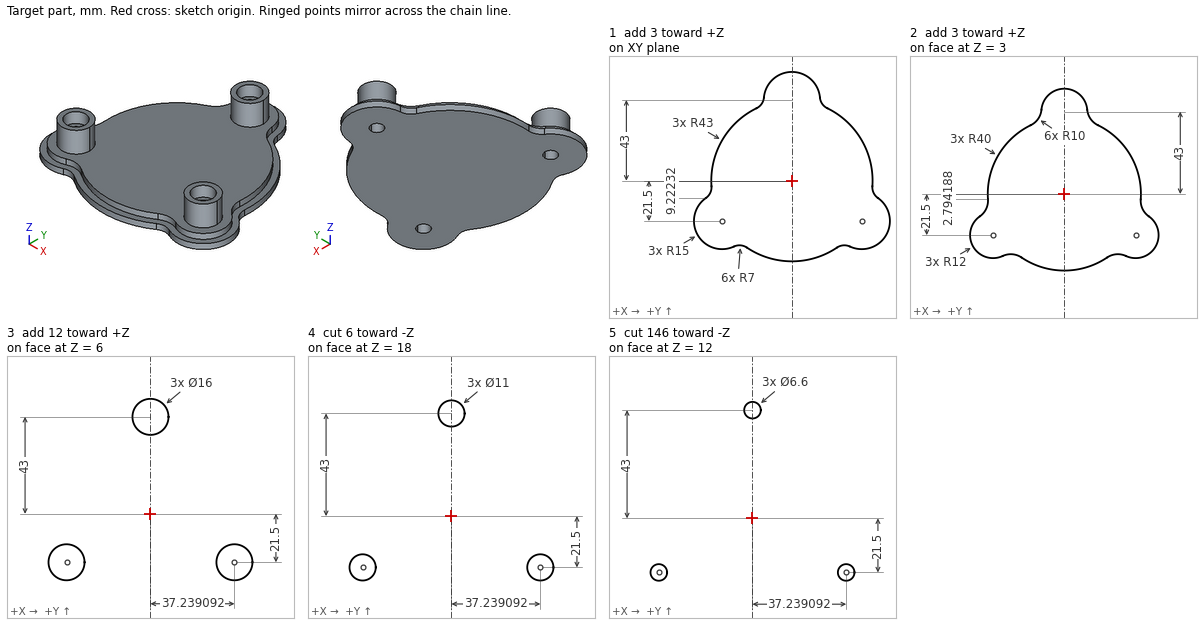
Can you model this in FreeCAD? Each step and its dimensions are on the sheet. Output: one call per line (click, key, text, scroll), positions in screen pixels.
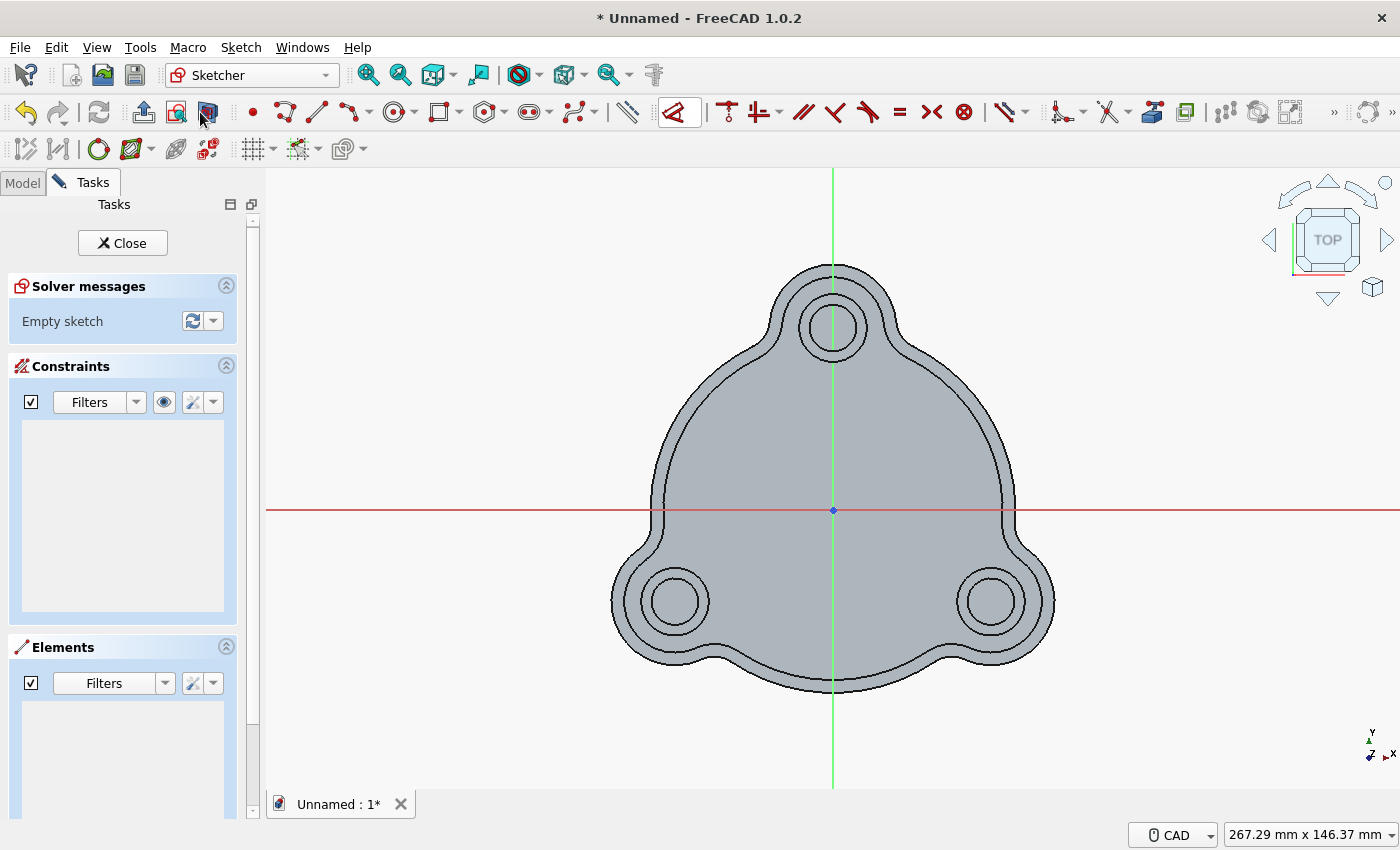
click(208, 112)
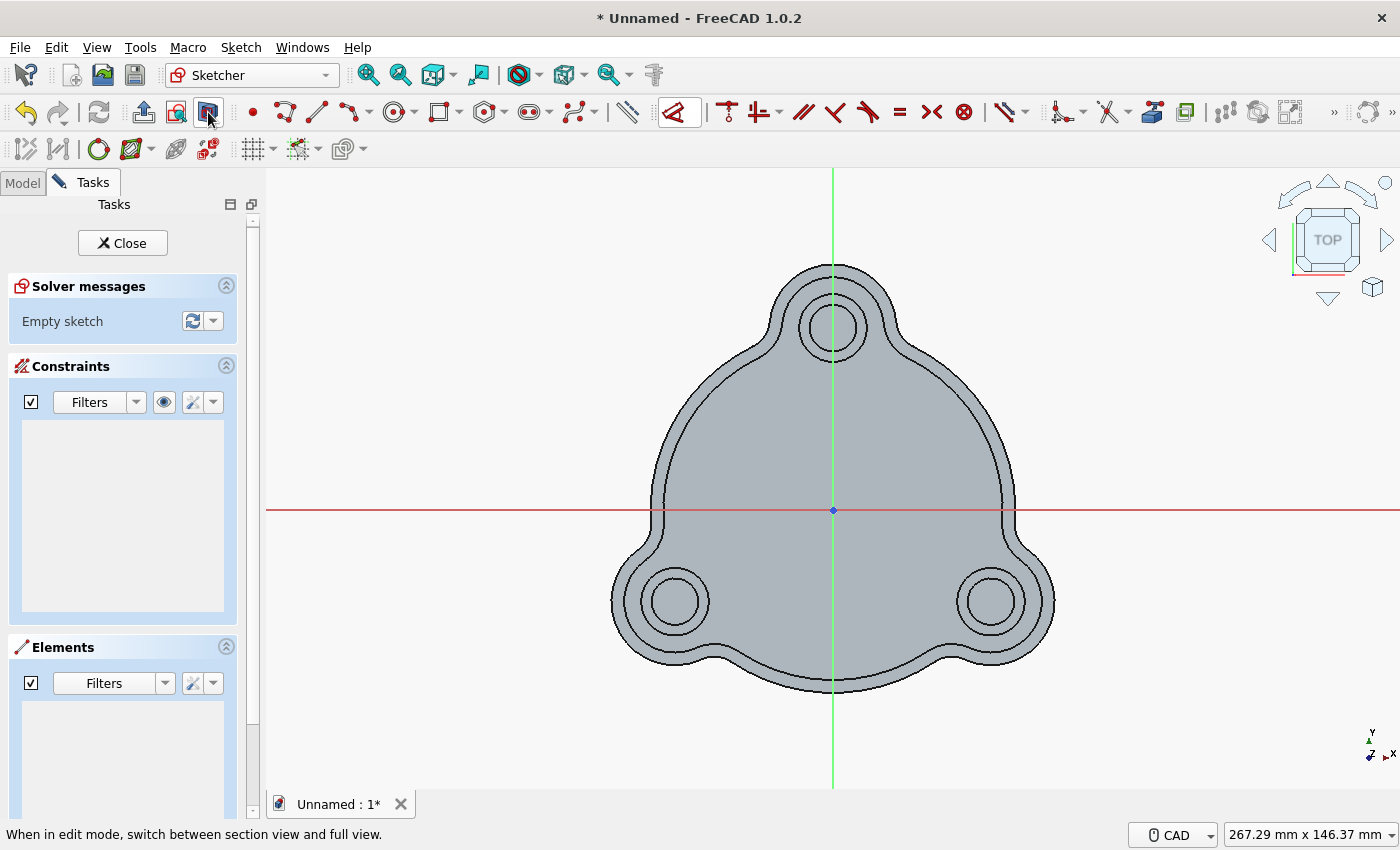
click(394, 112)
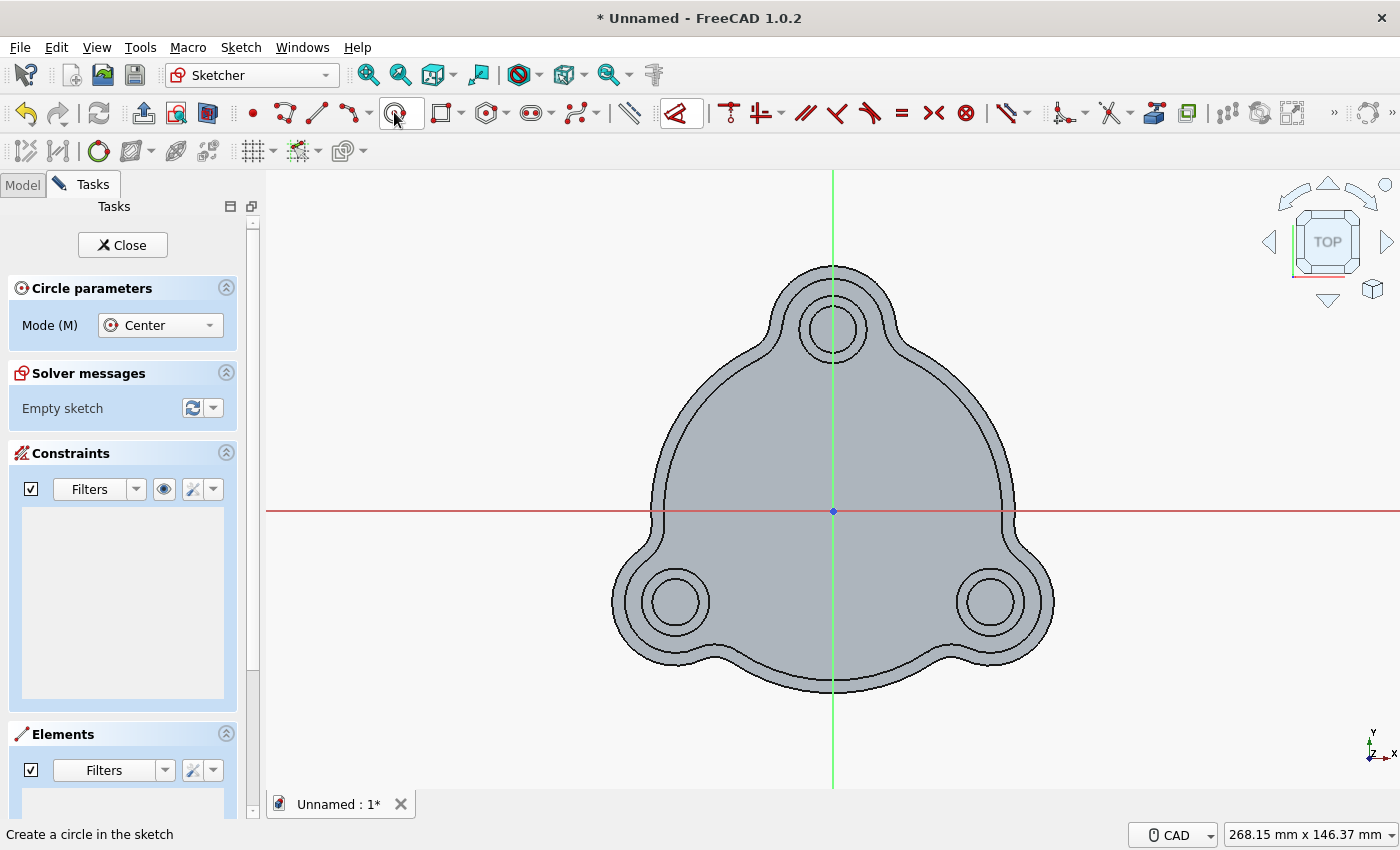
scroll(833, 330, up, 3)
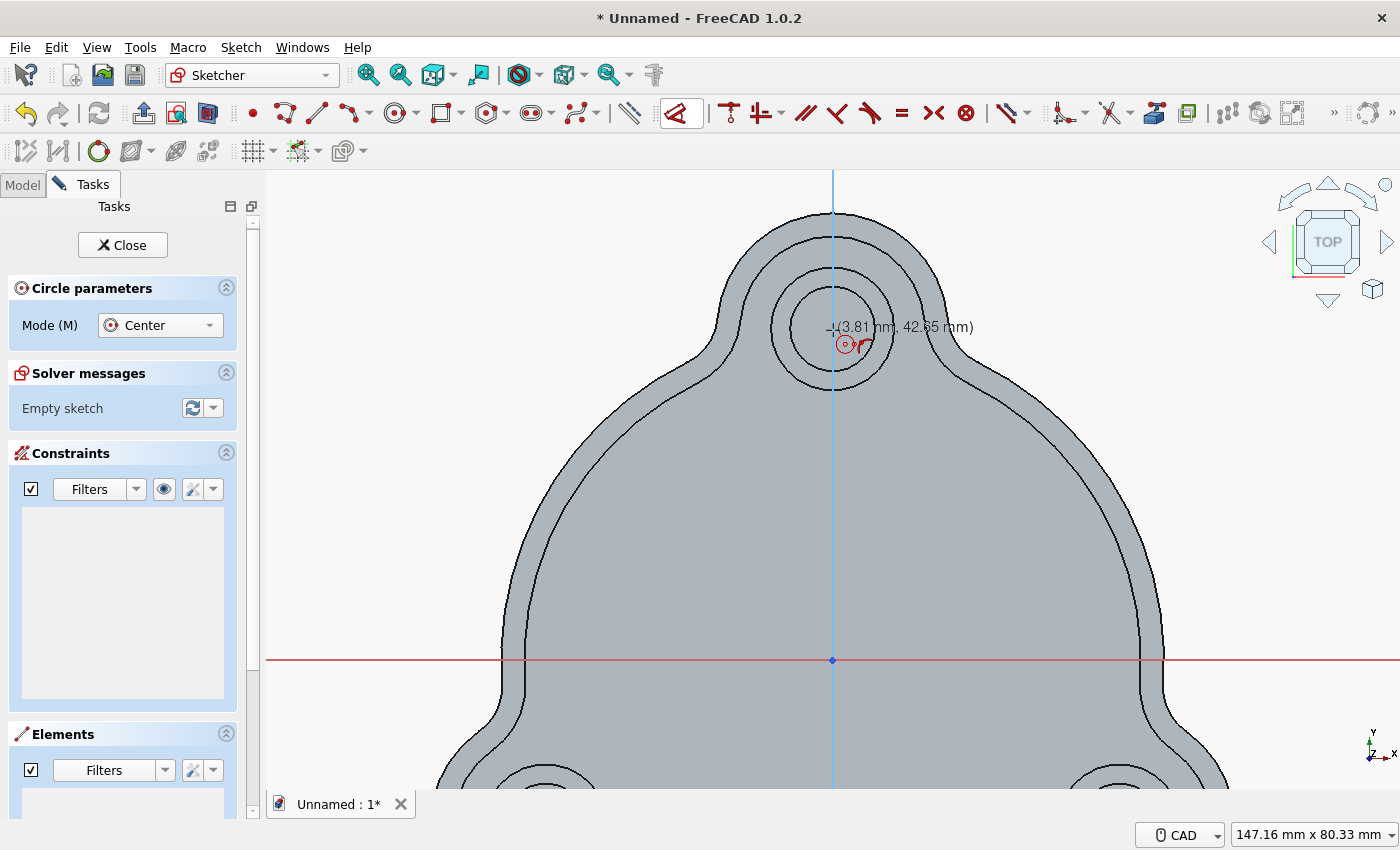
click(833, 329)
move(851, 311)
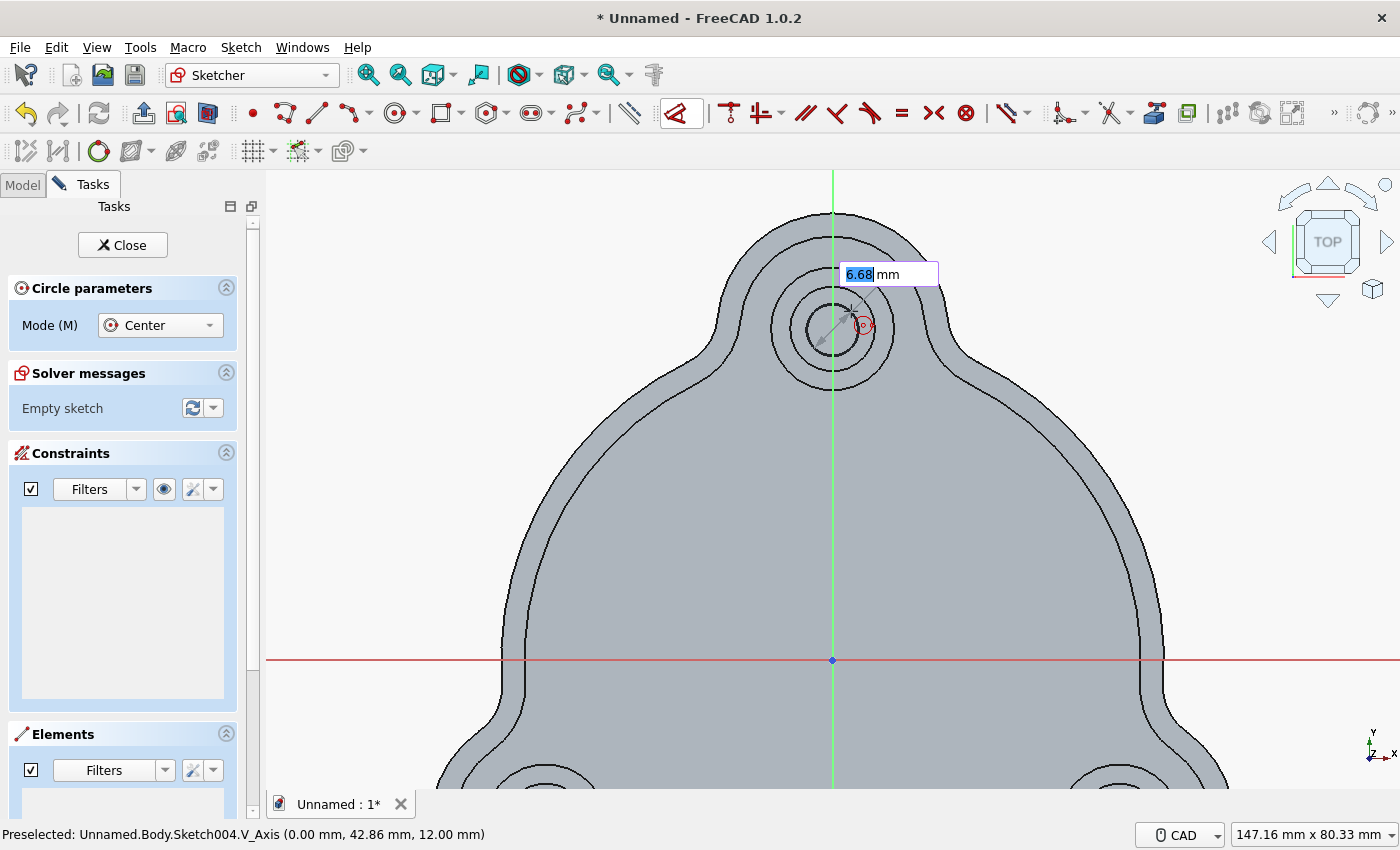
text(6.6)
key(Return)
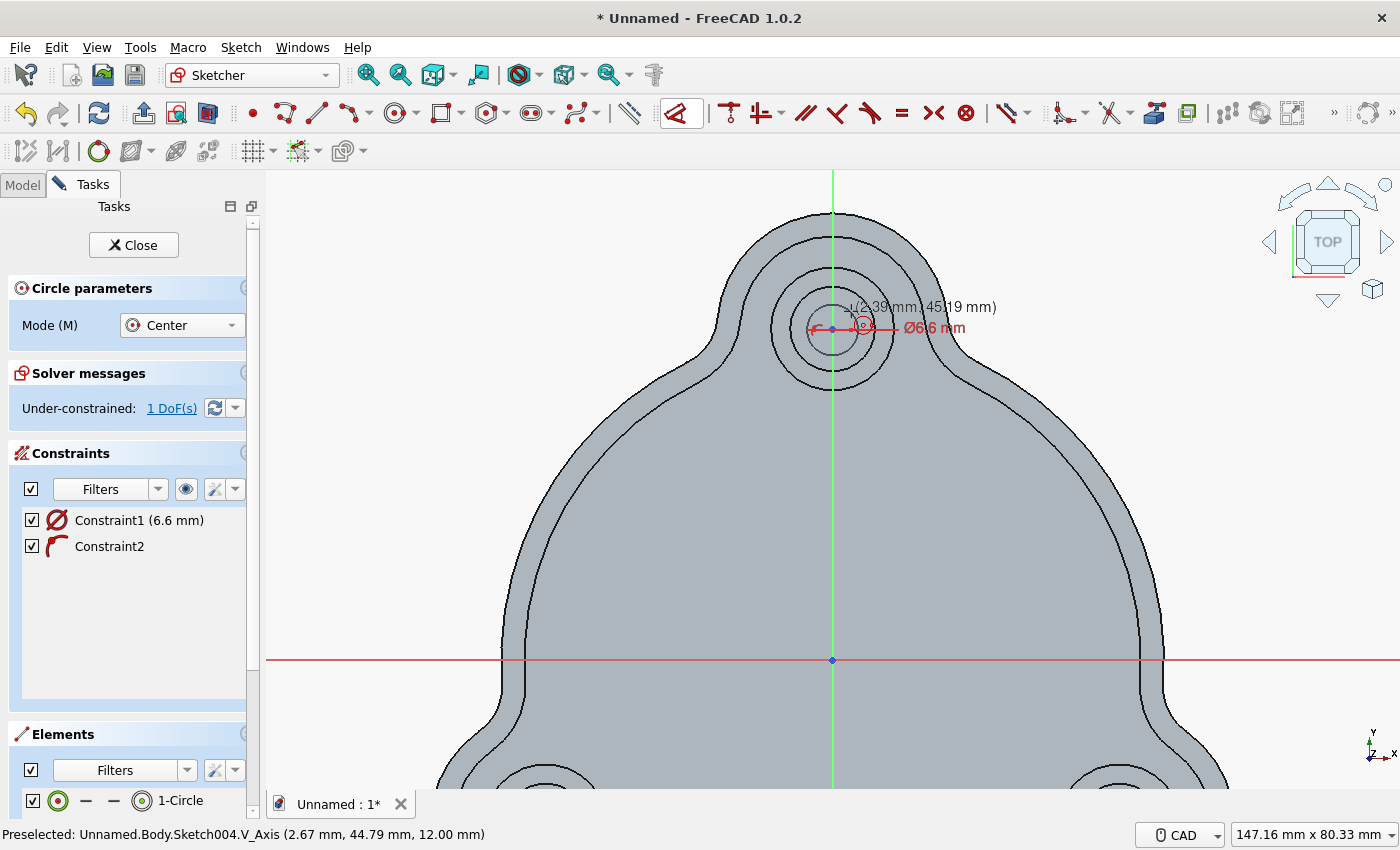
scroll(626, 280, down, 2)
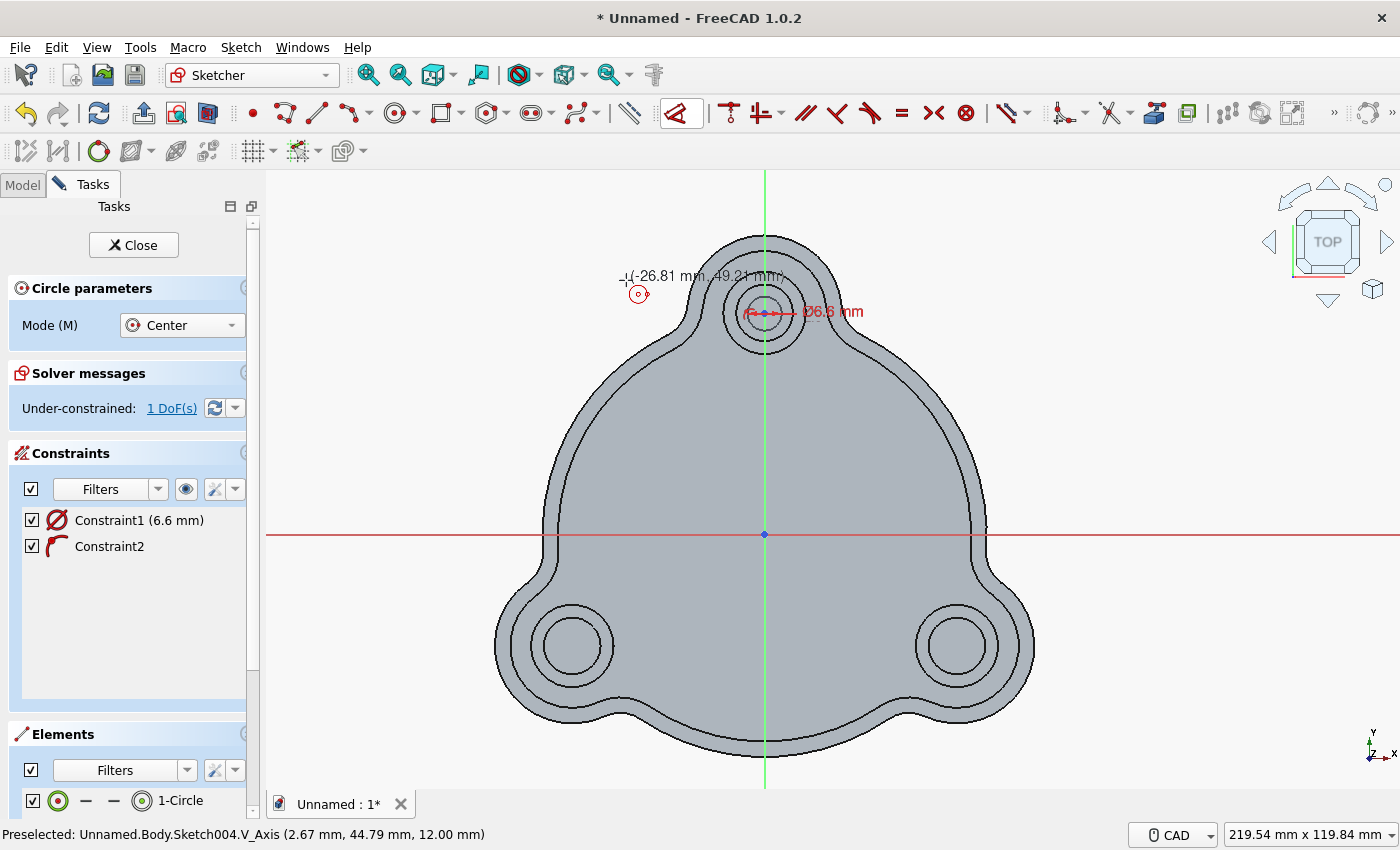
scroll(957, 646, up, 2)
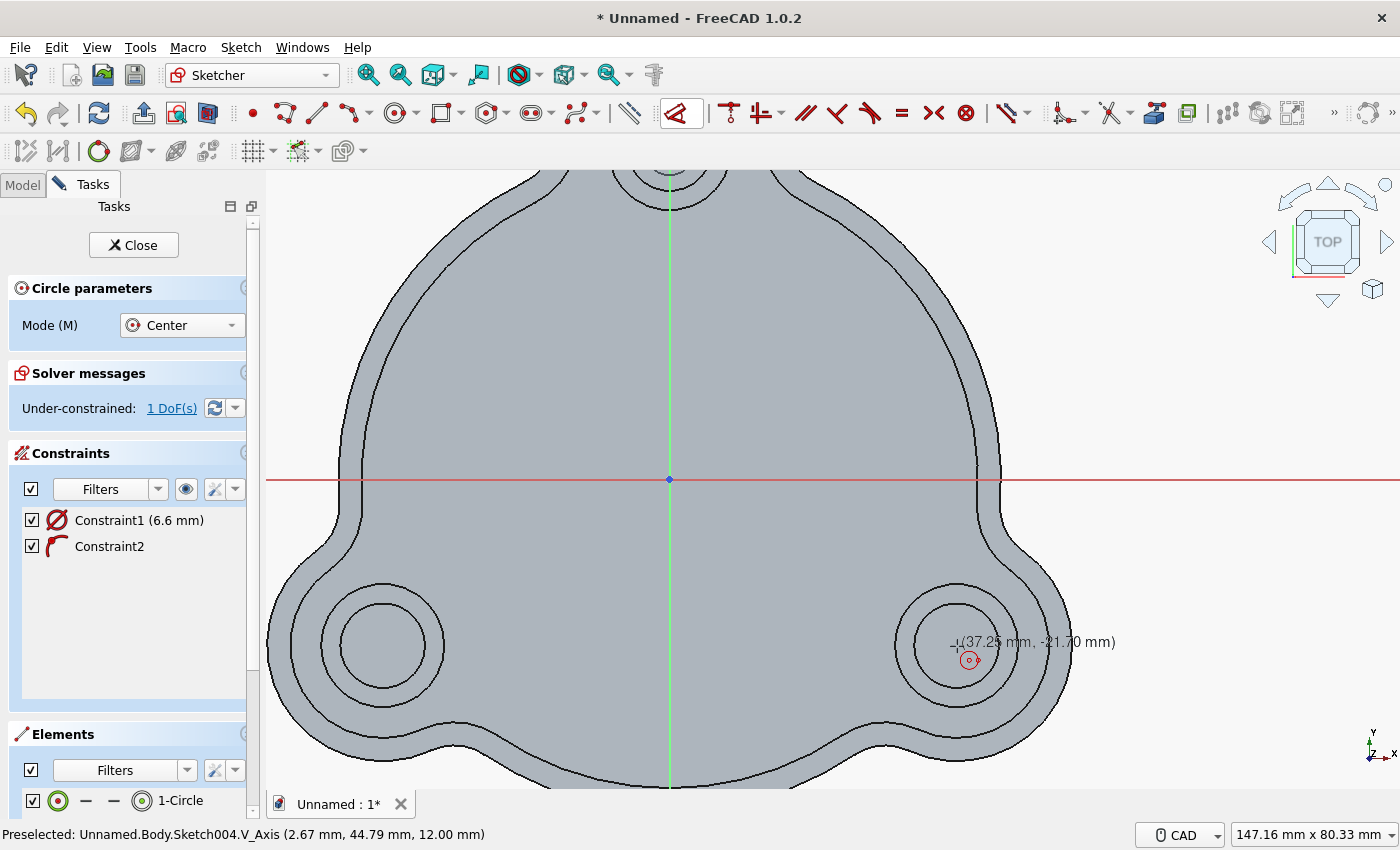
click(957, 646)
move(975, 628)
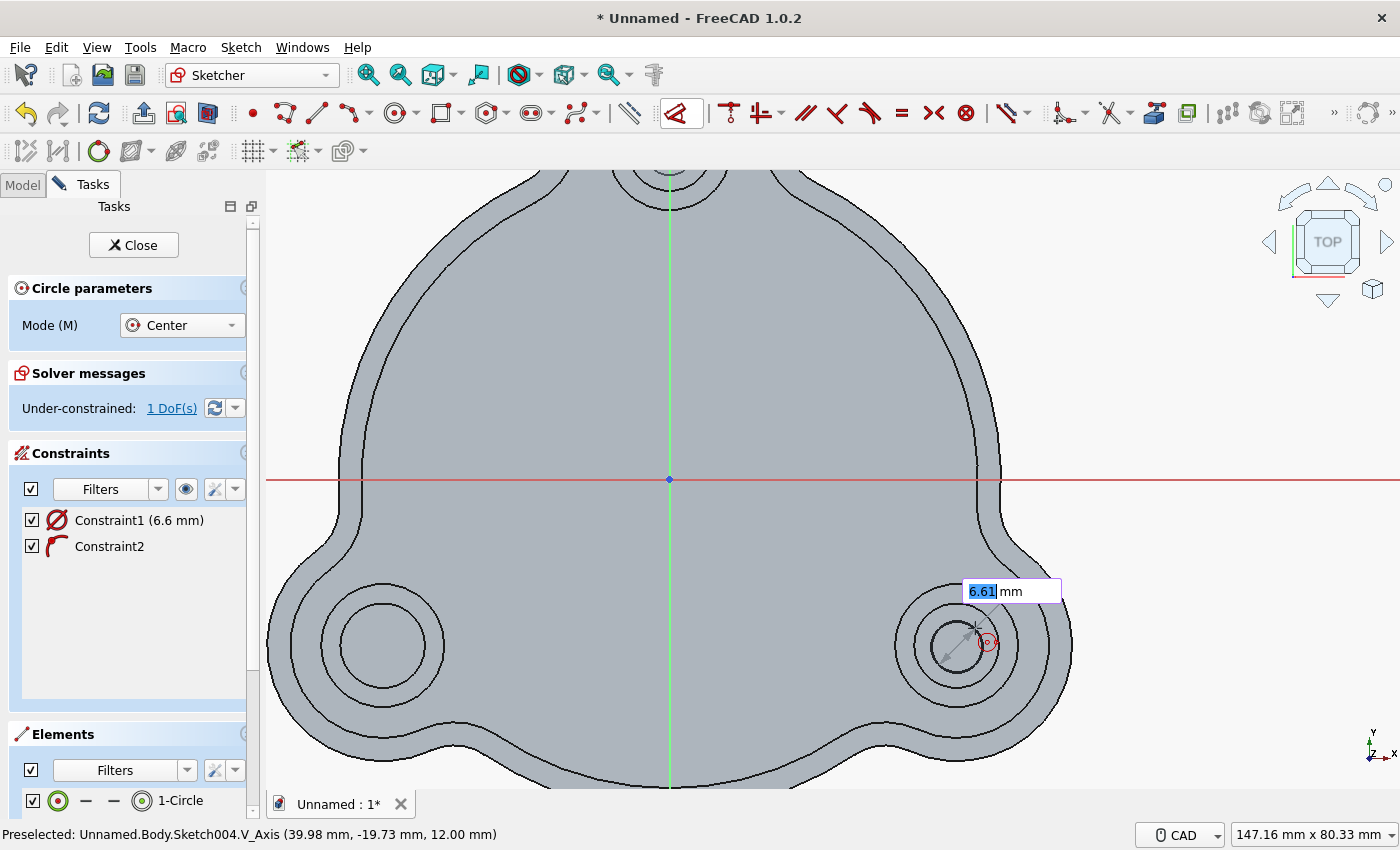
text(6.6)
key(Return)